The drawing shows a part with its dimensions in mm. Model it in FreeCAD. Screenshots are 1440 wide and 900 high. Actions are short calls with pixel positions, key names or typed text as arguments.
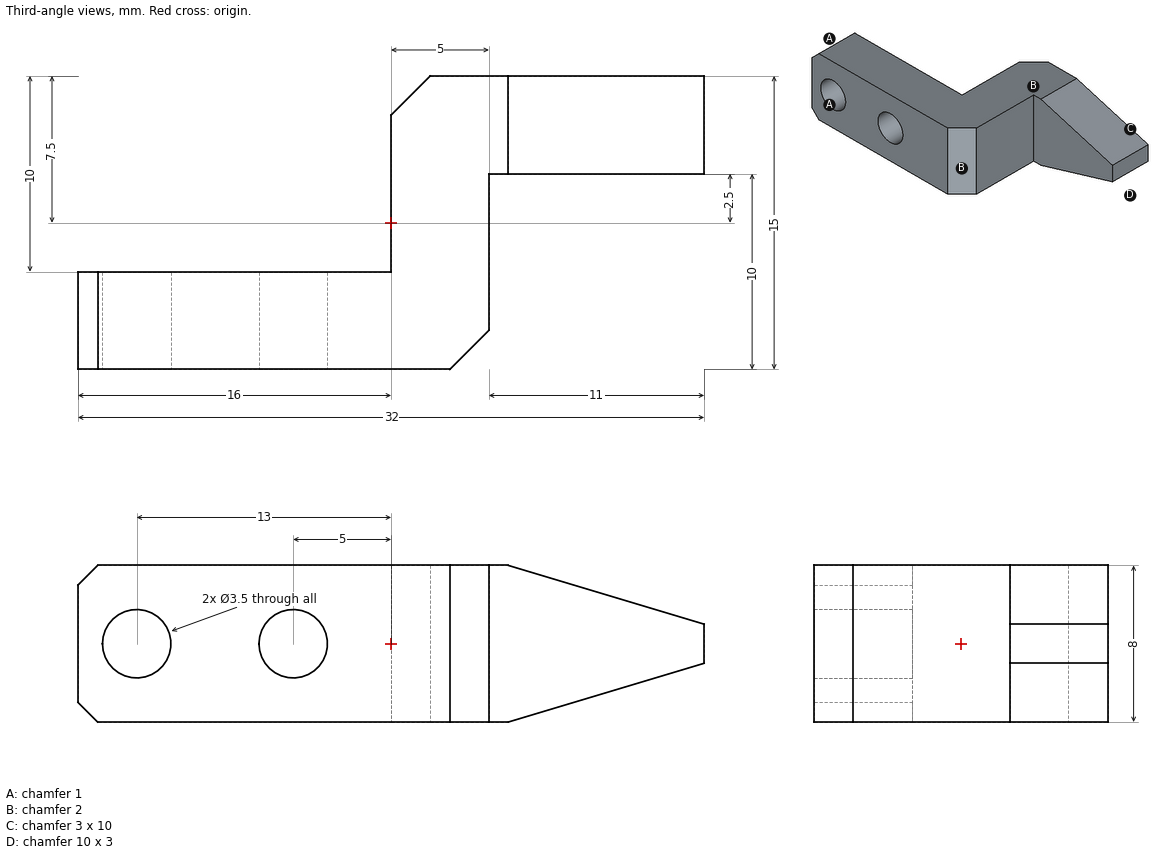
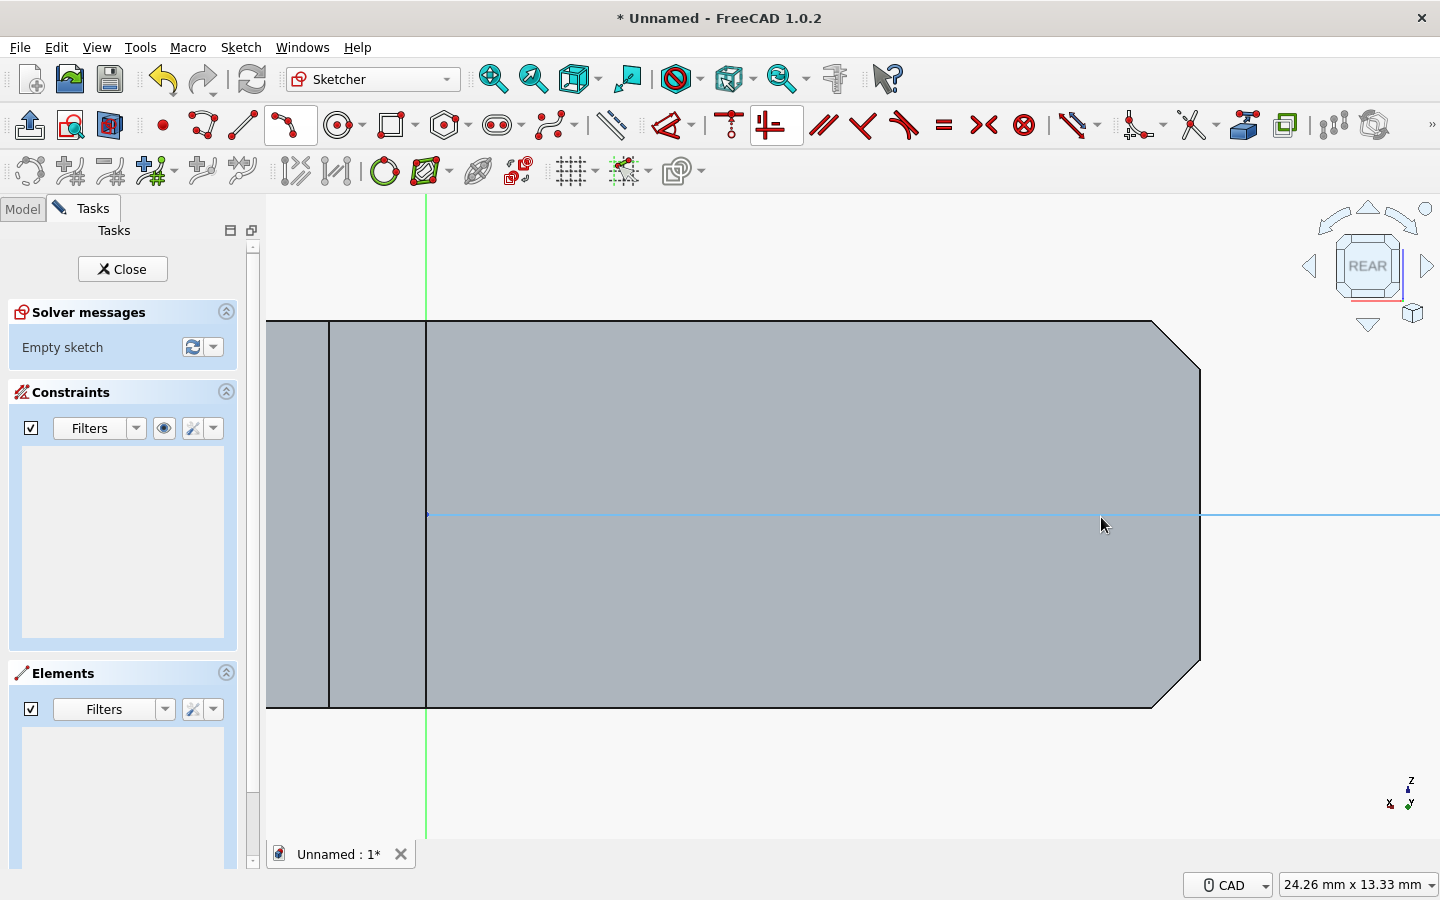
key(g)
key(c)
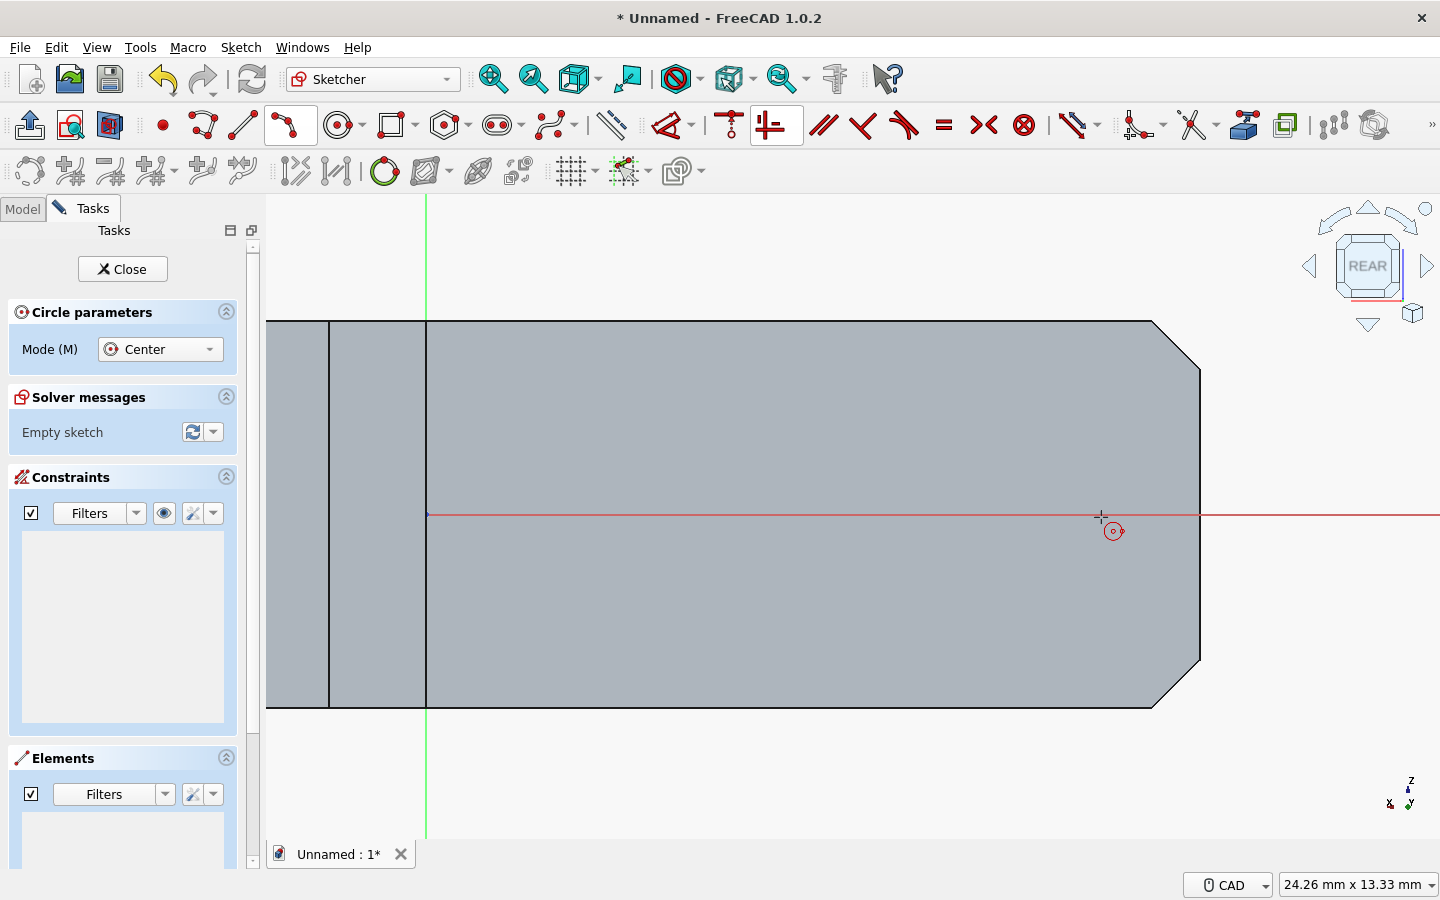
click(1055, 515)
move(1115, 455)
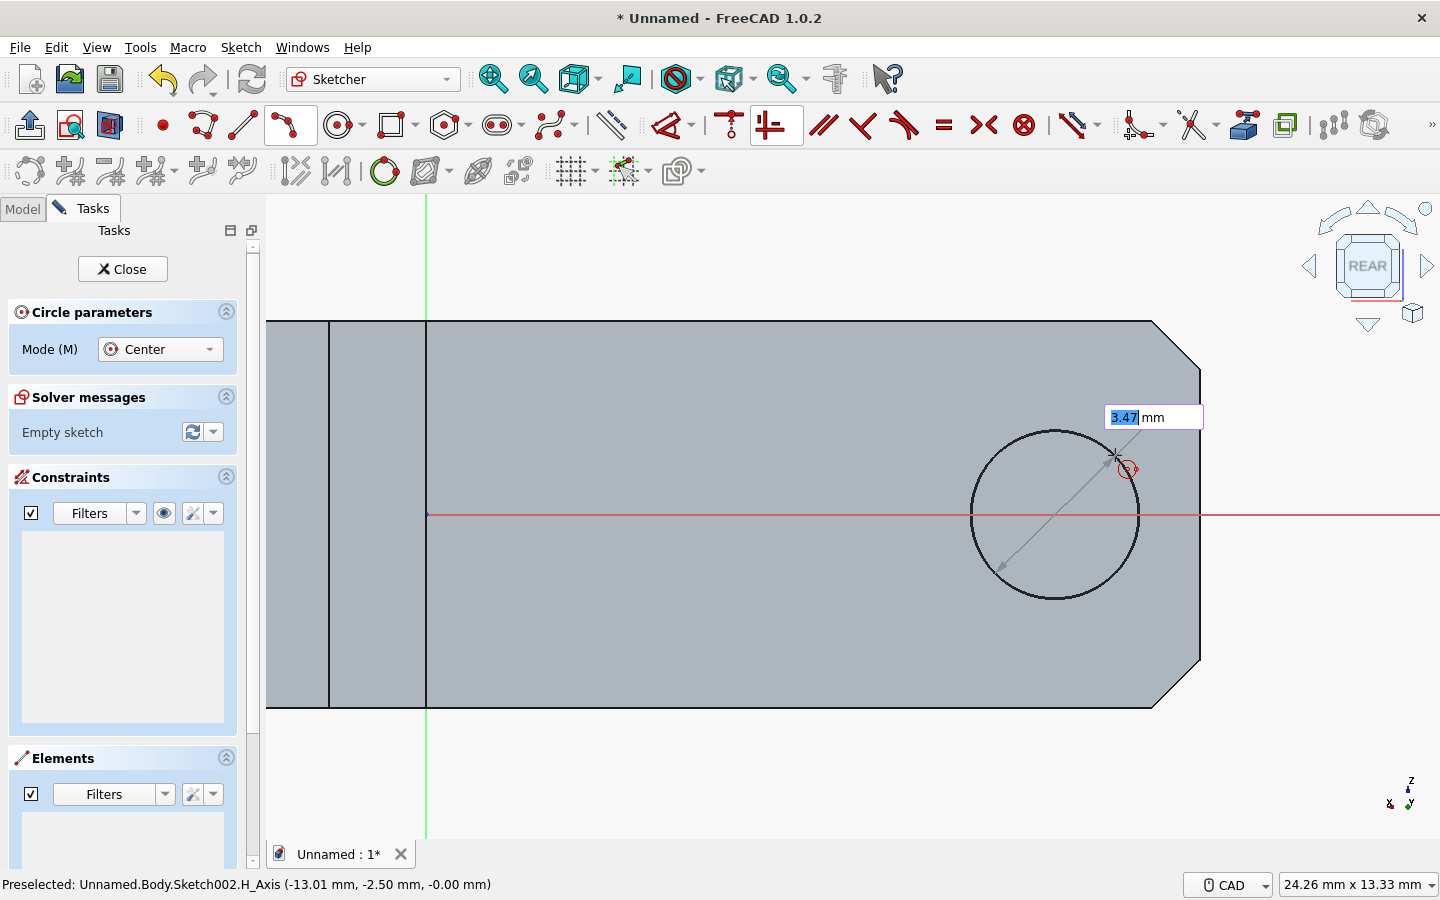
text(3.5)
key(Return)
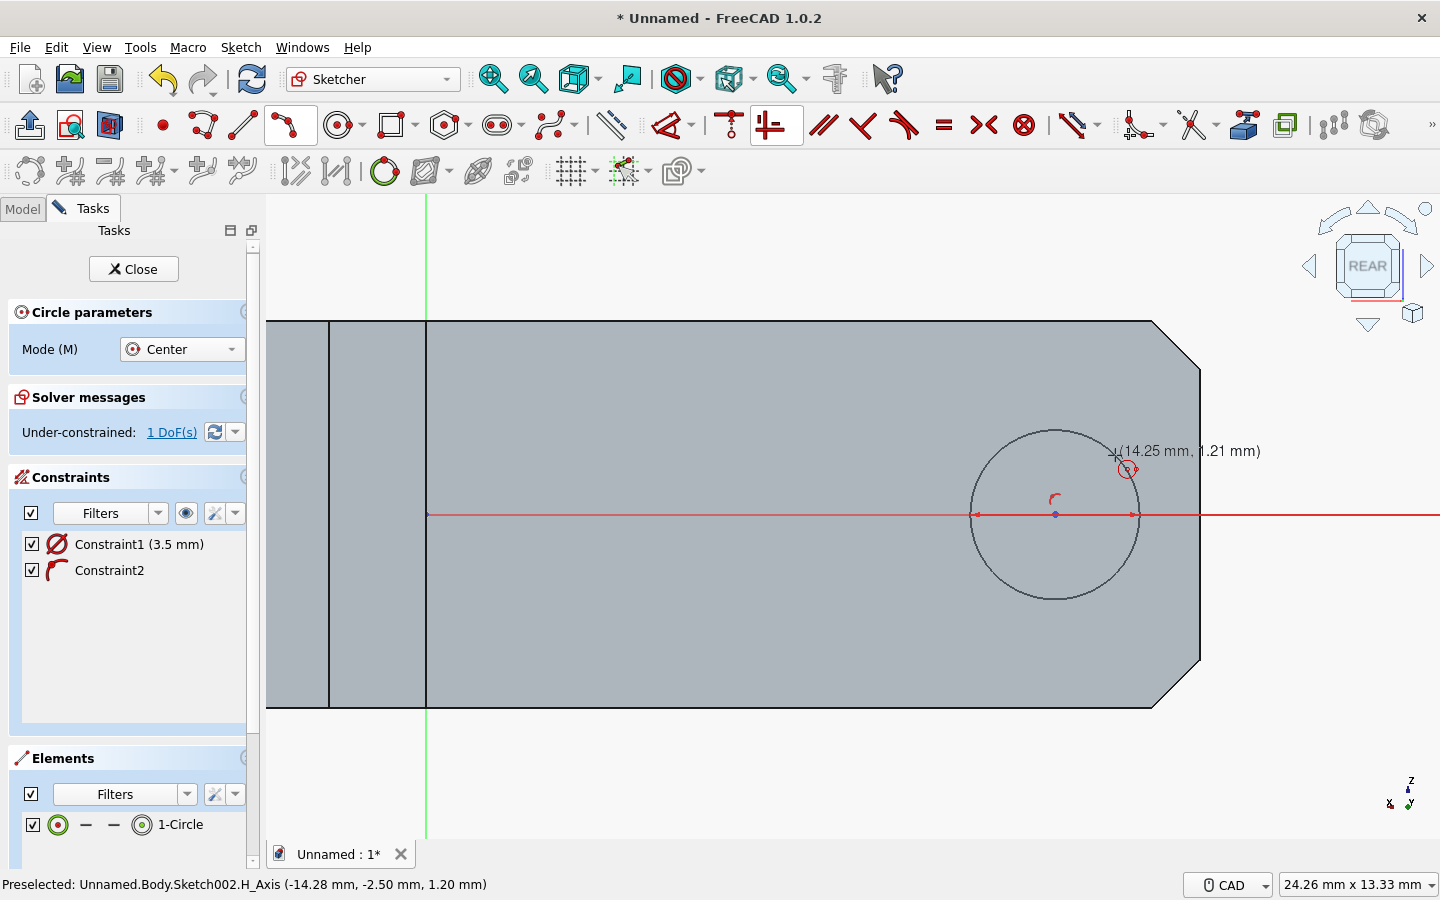
click(668, 515)
move(727, 455)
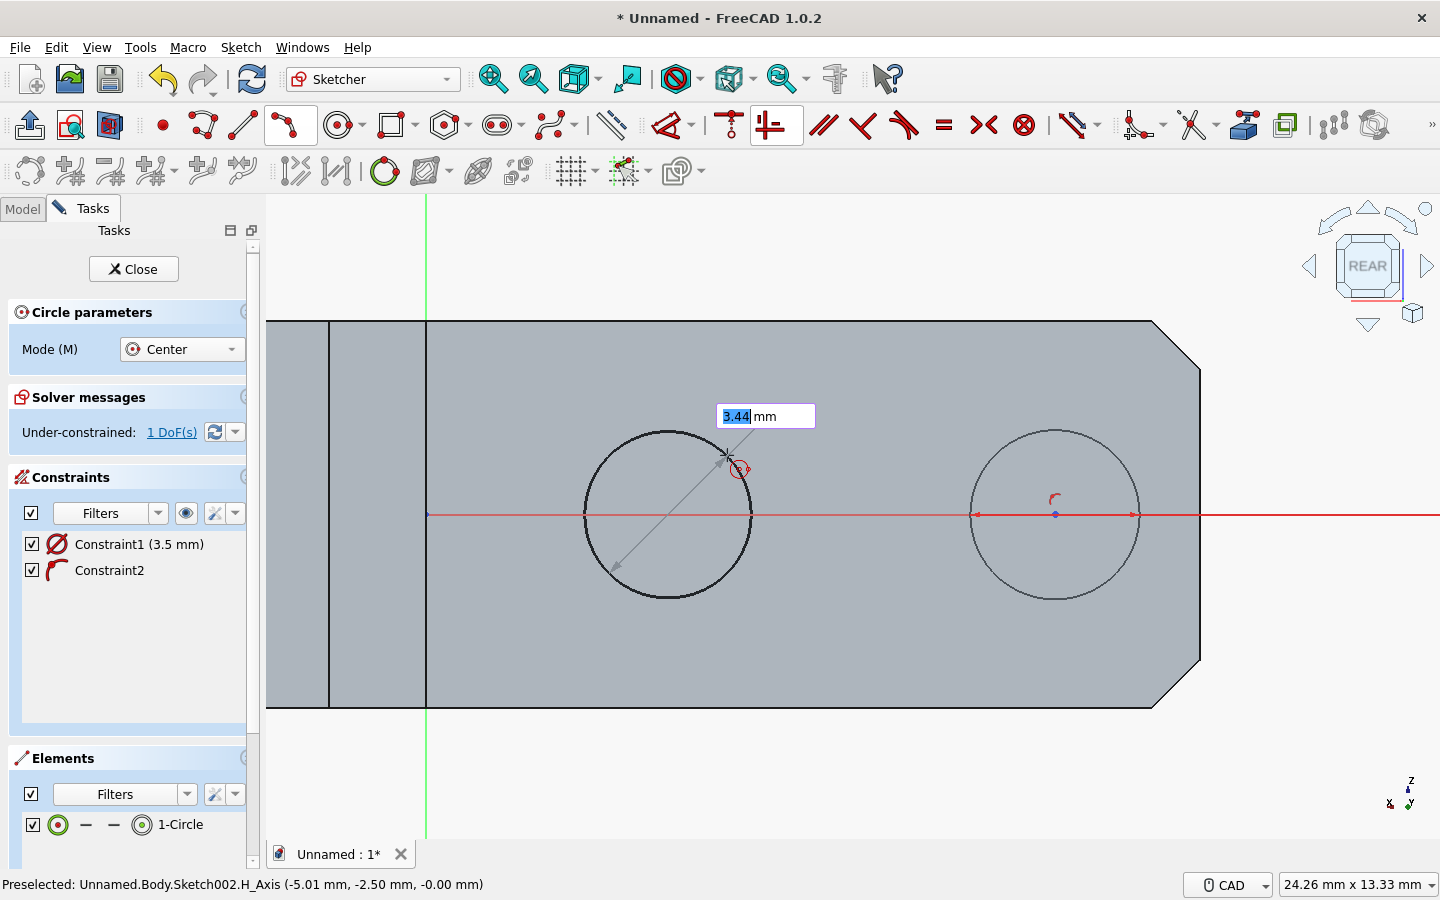
text(3.5)
key(Return)
key(Escape)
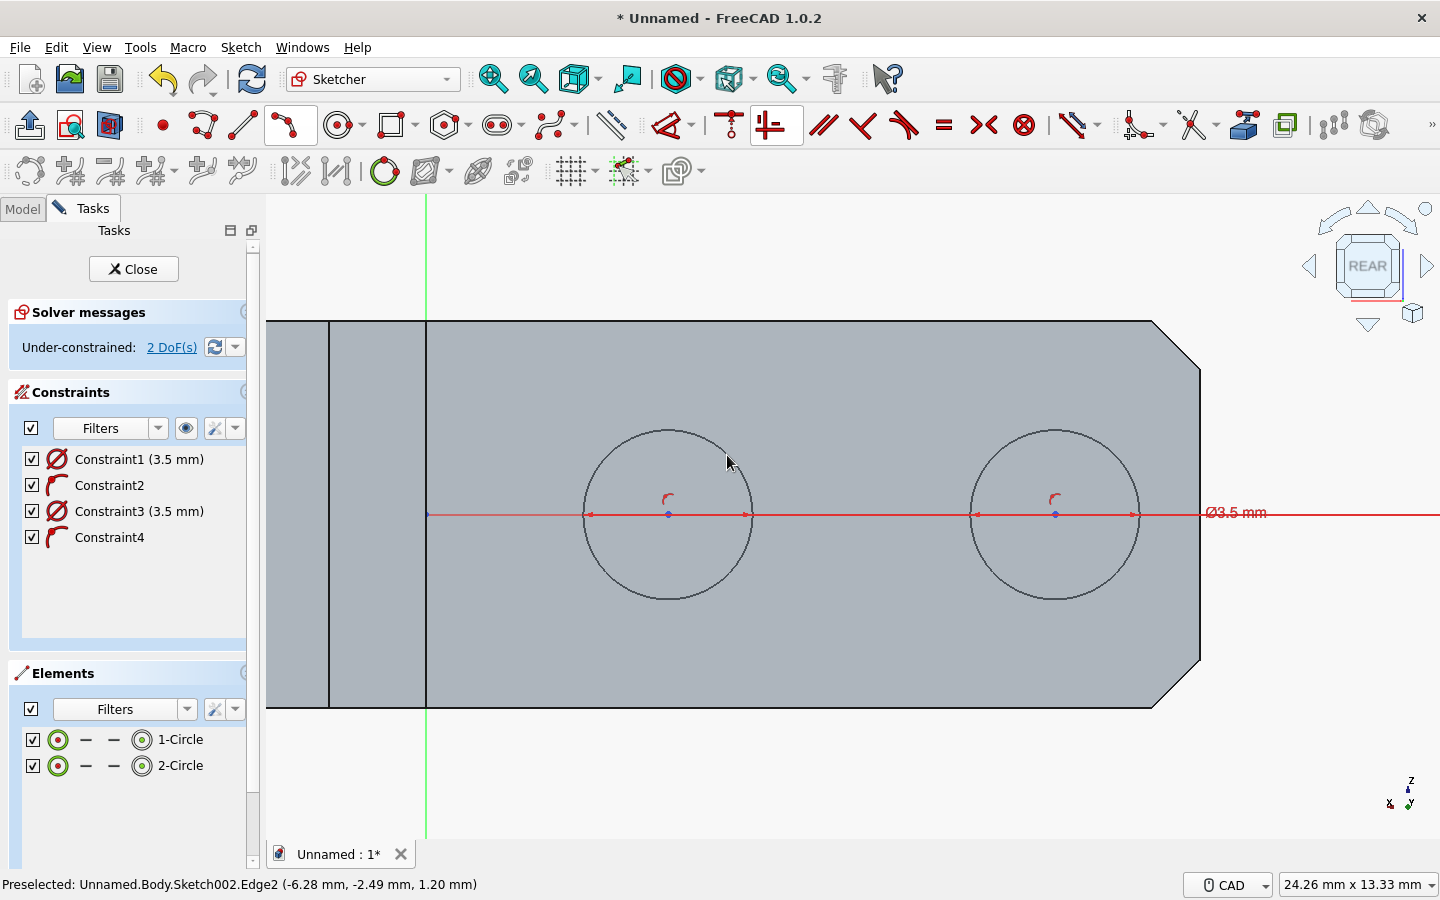
key(d)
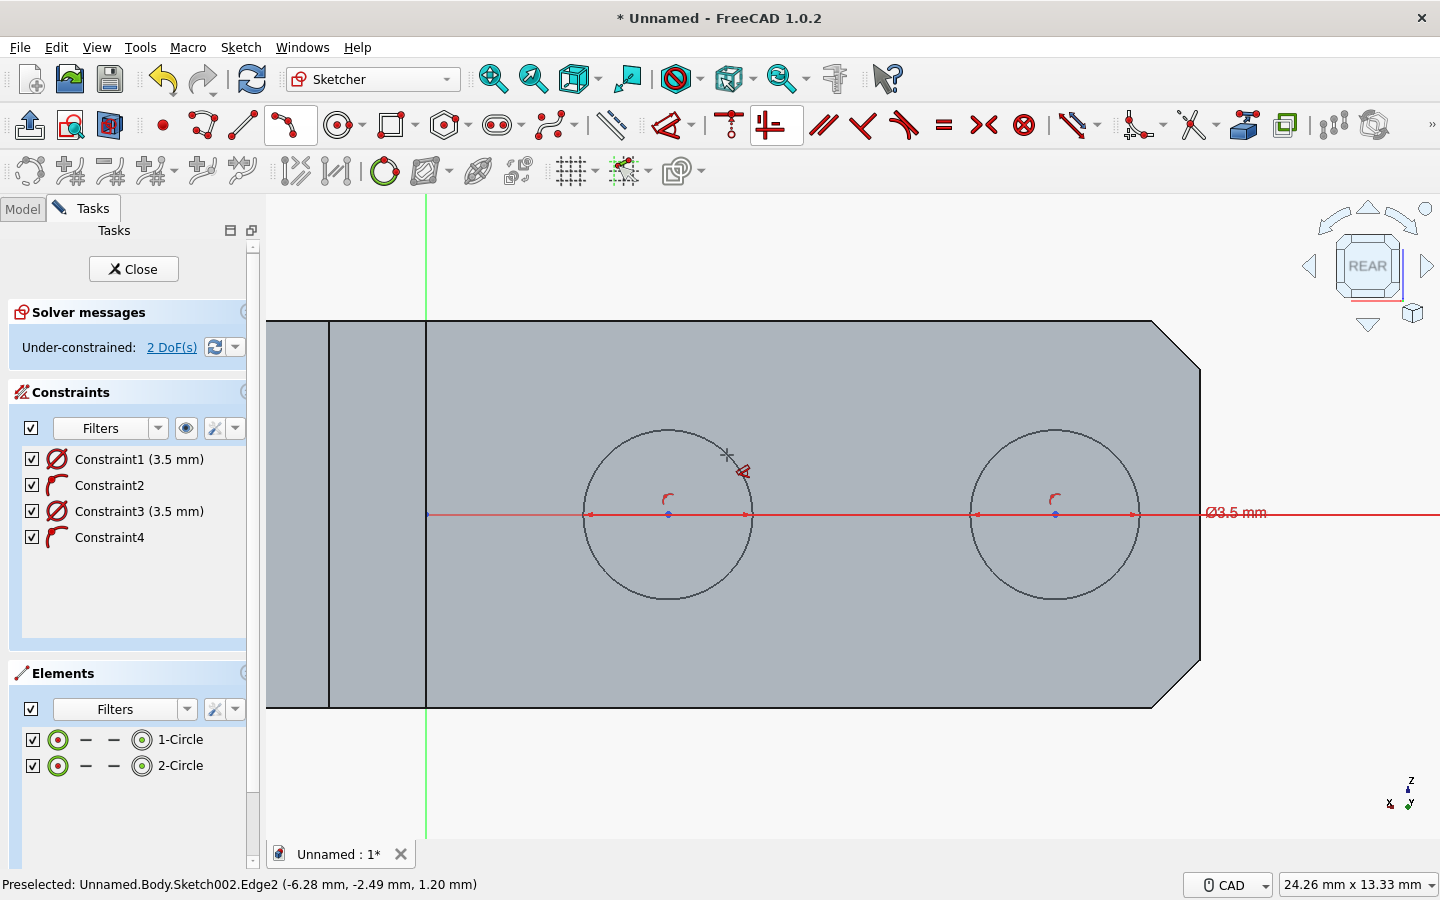
click(668, 515)
click(547, 549)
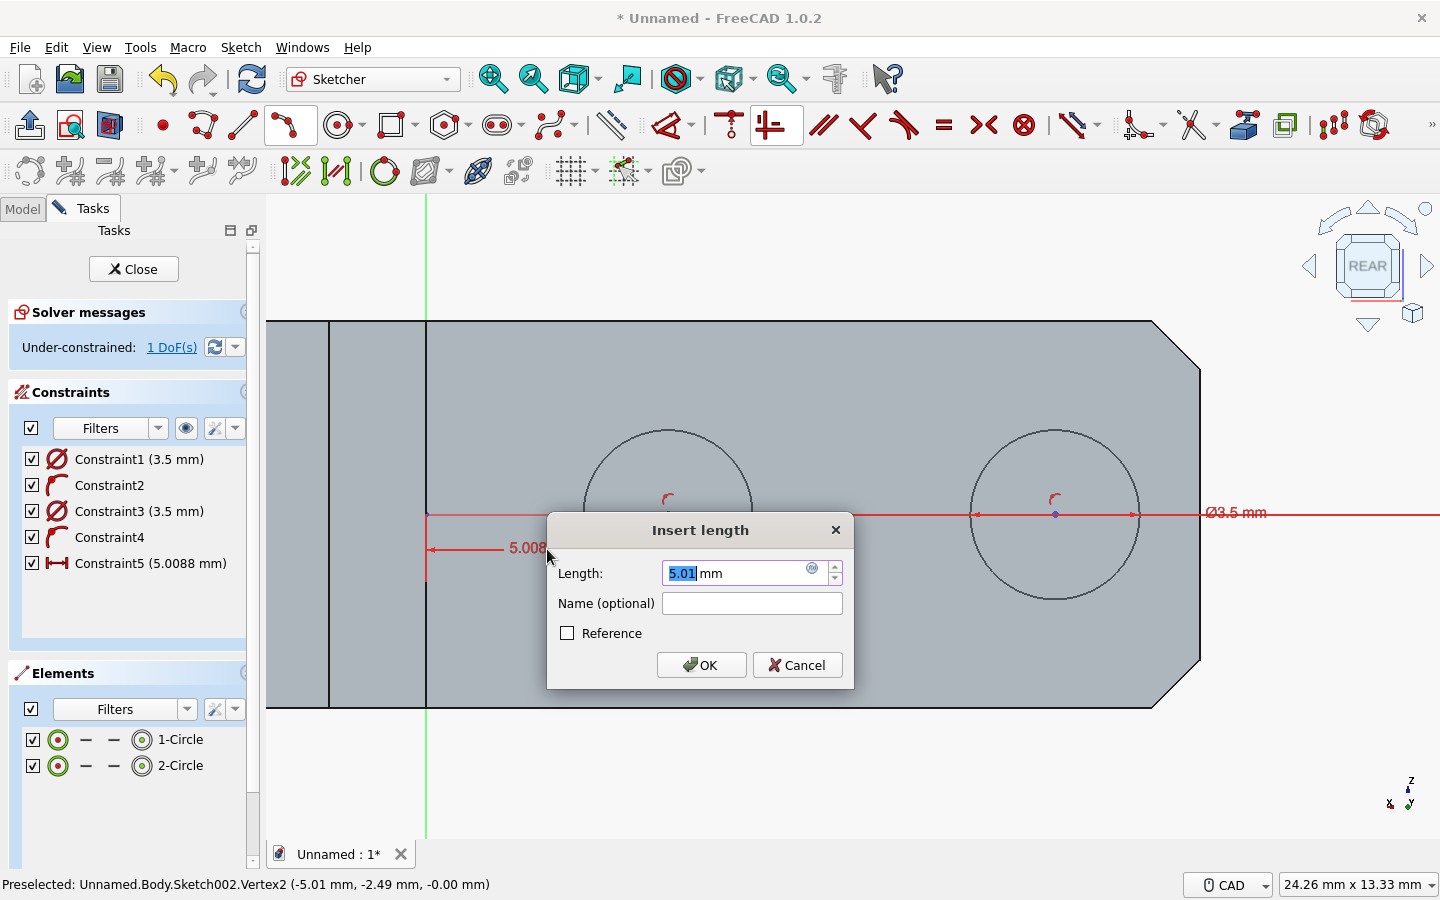
text(5)
key(Return)